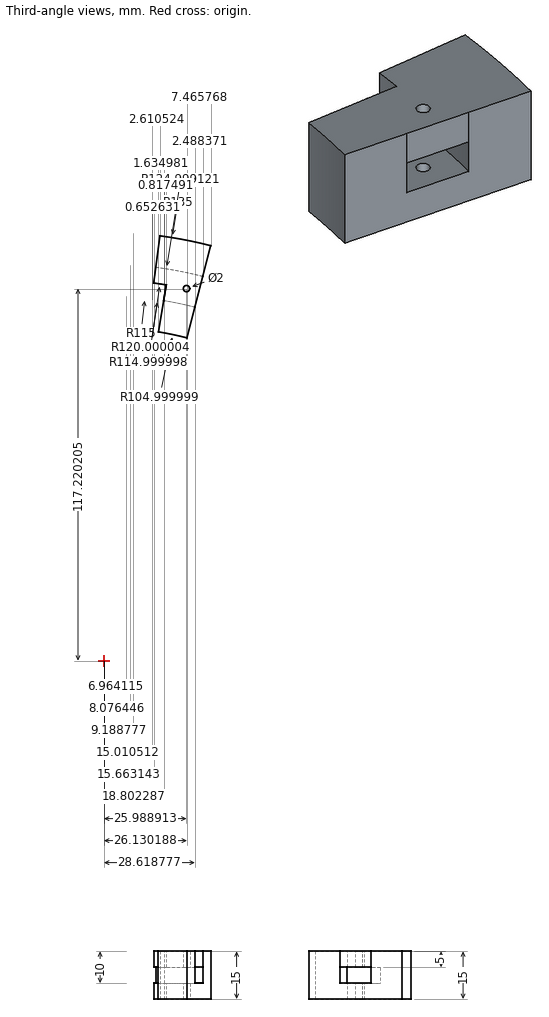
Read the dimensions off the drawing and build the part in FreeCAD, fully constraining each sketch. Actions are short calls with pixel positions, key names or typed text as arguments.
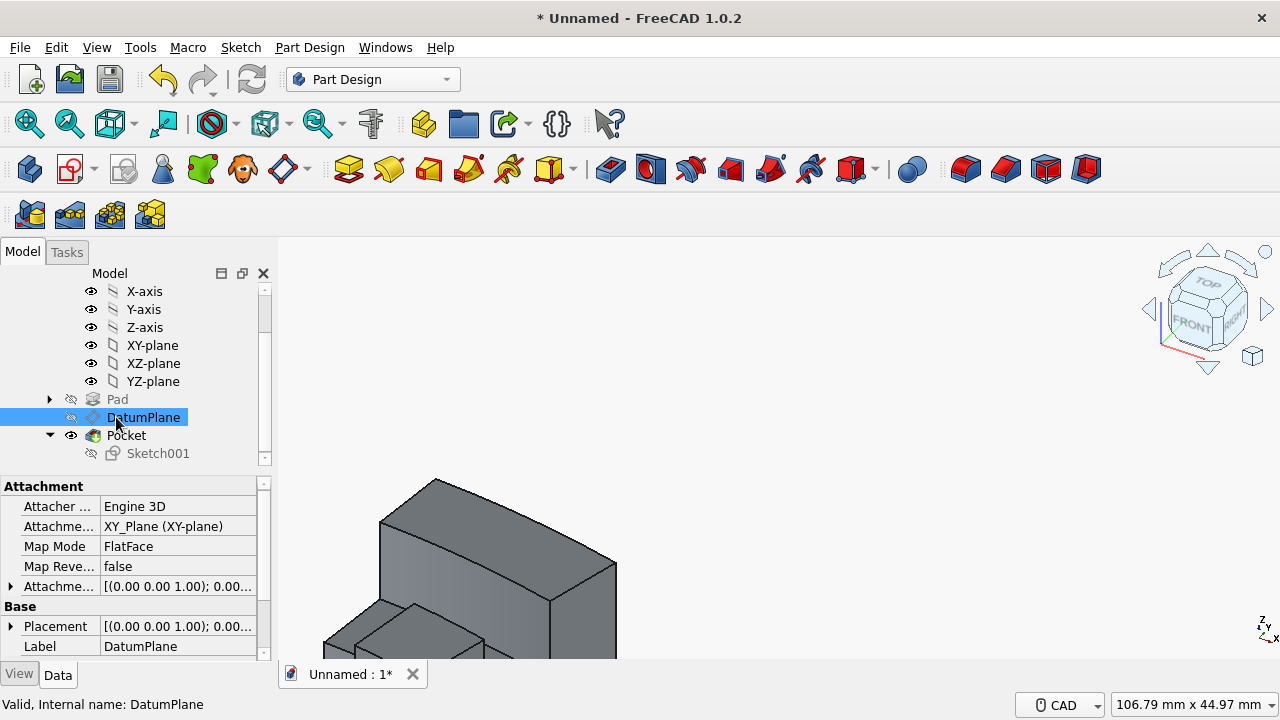
click(30, 124)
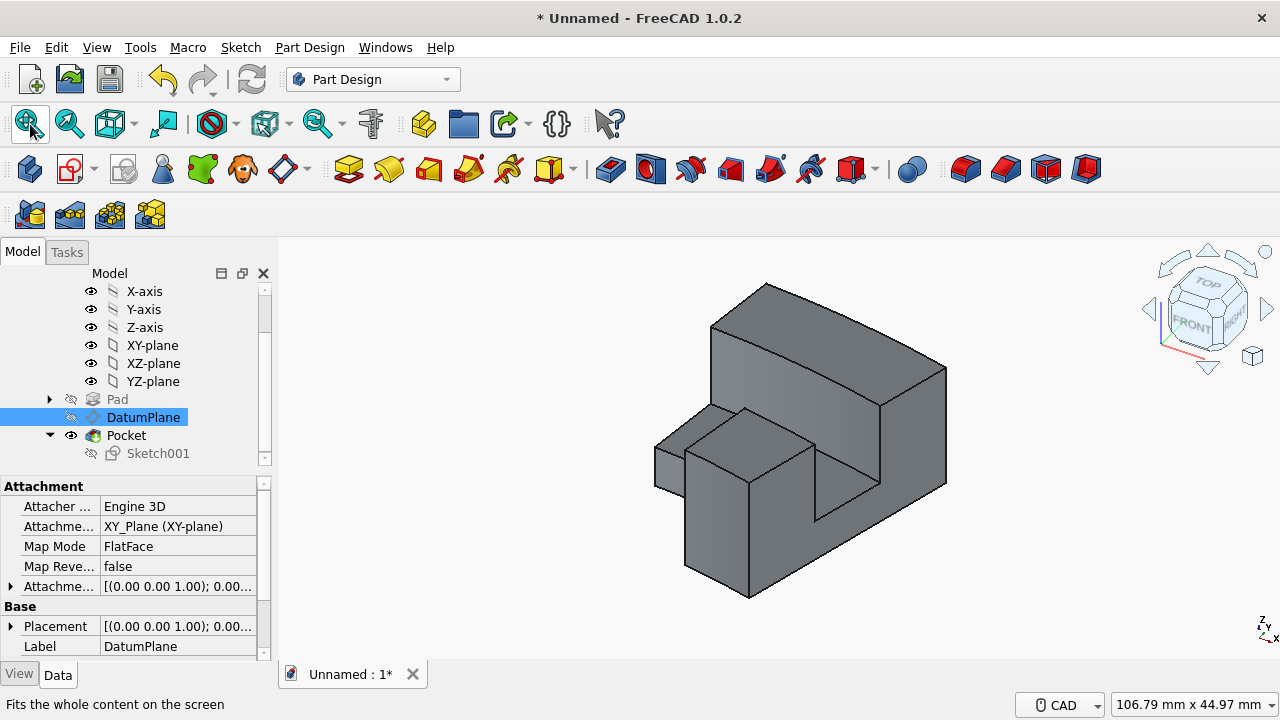
scroll(160, 377, down, 3)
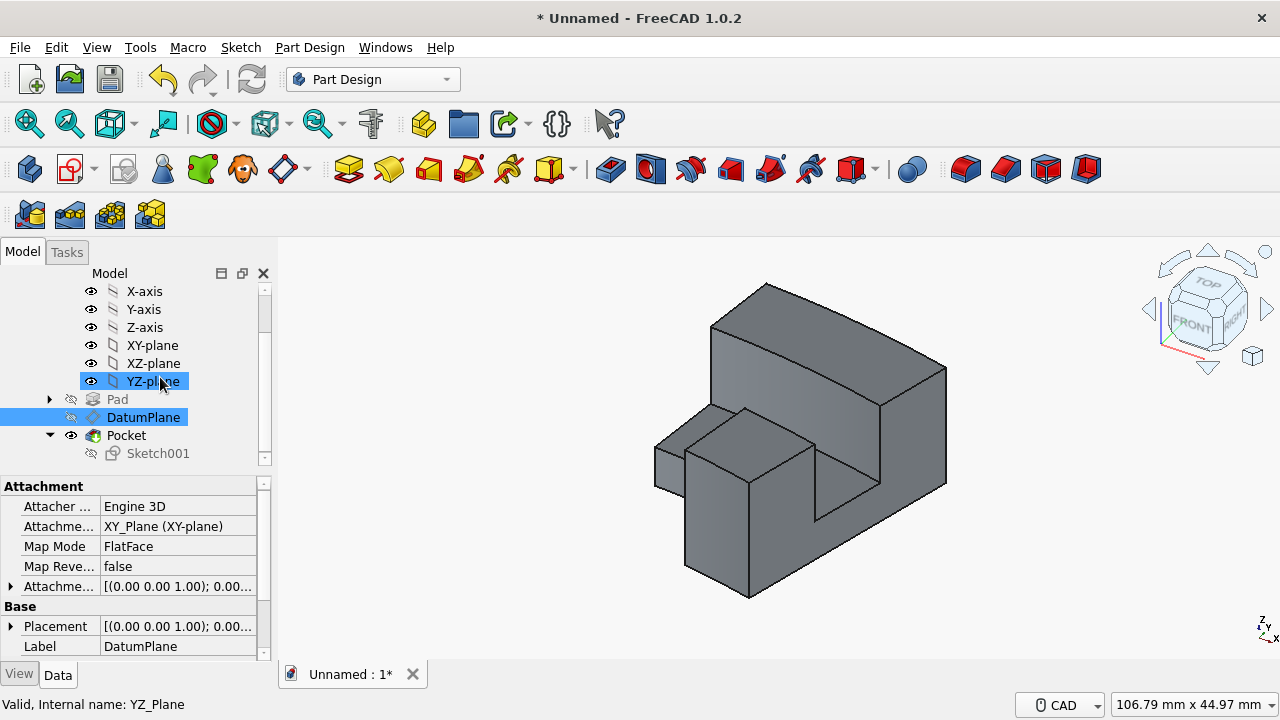
scroll(160, 377, up, 15)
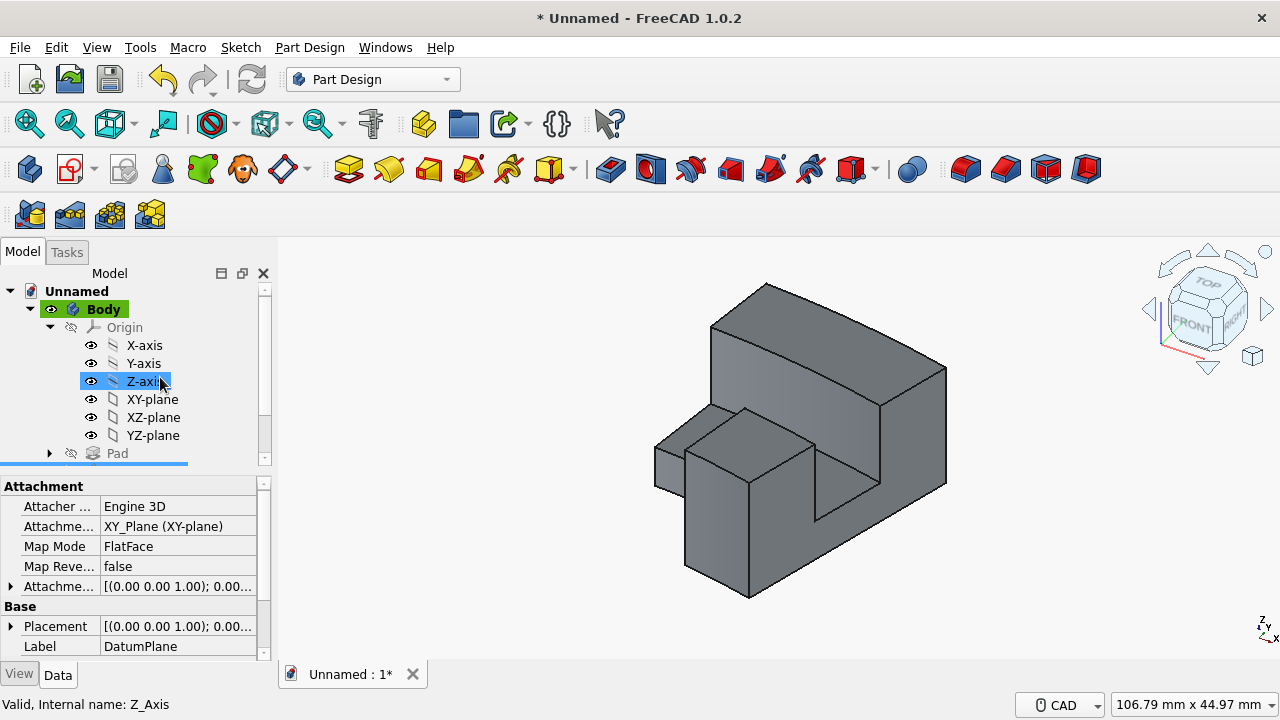
click(136, 399)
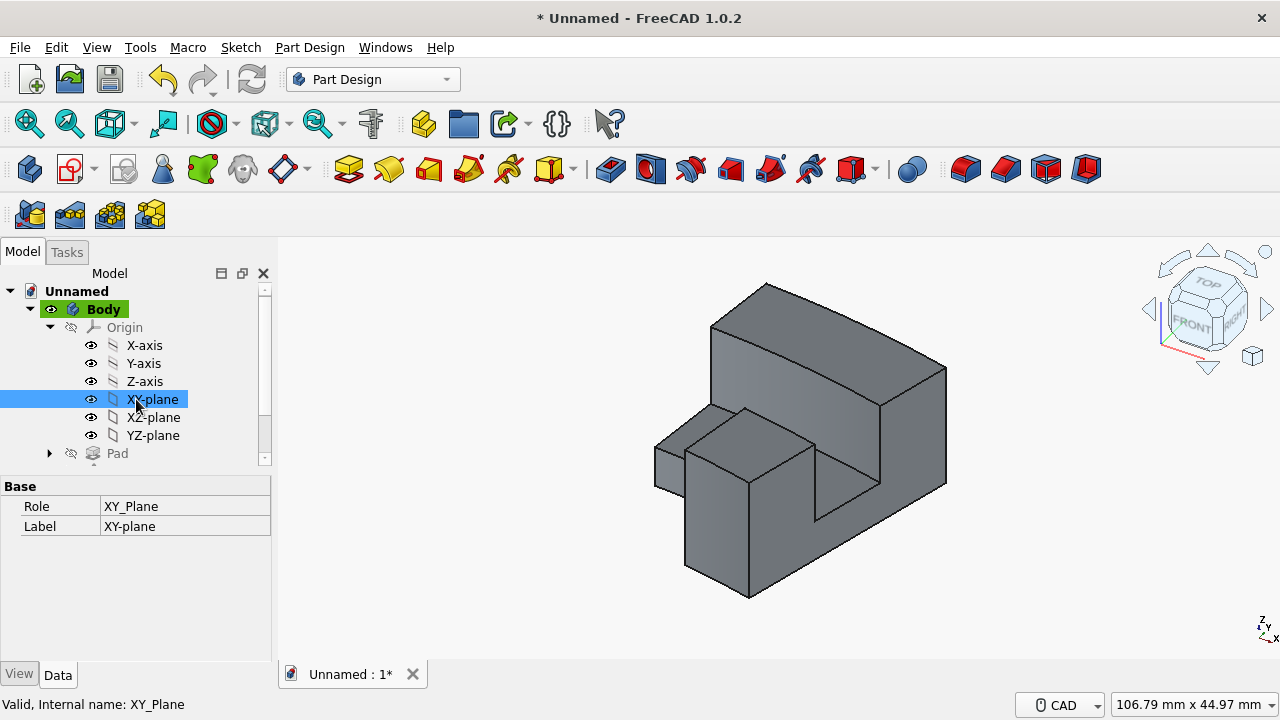
click(284, 170)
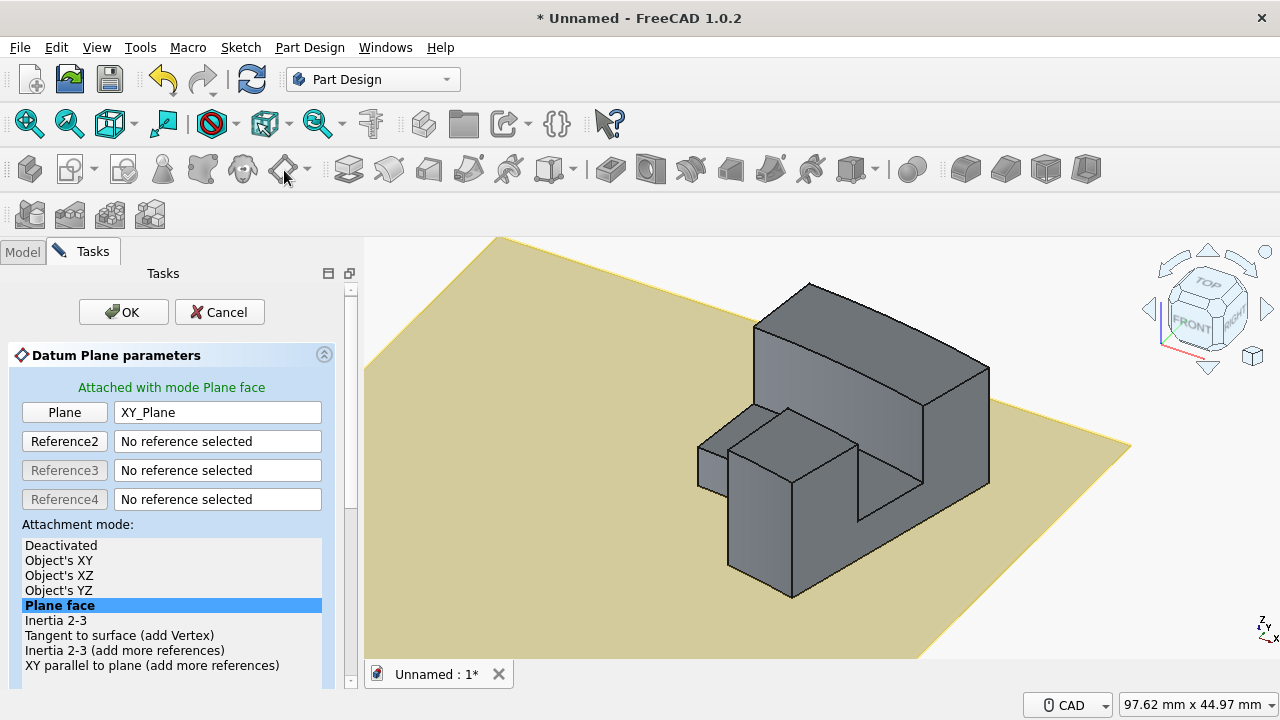
scroll(351, 486, down, 4)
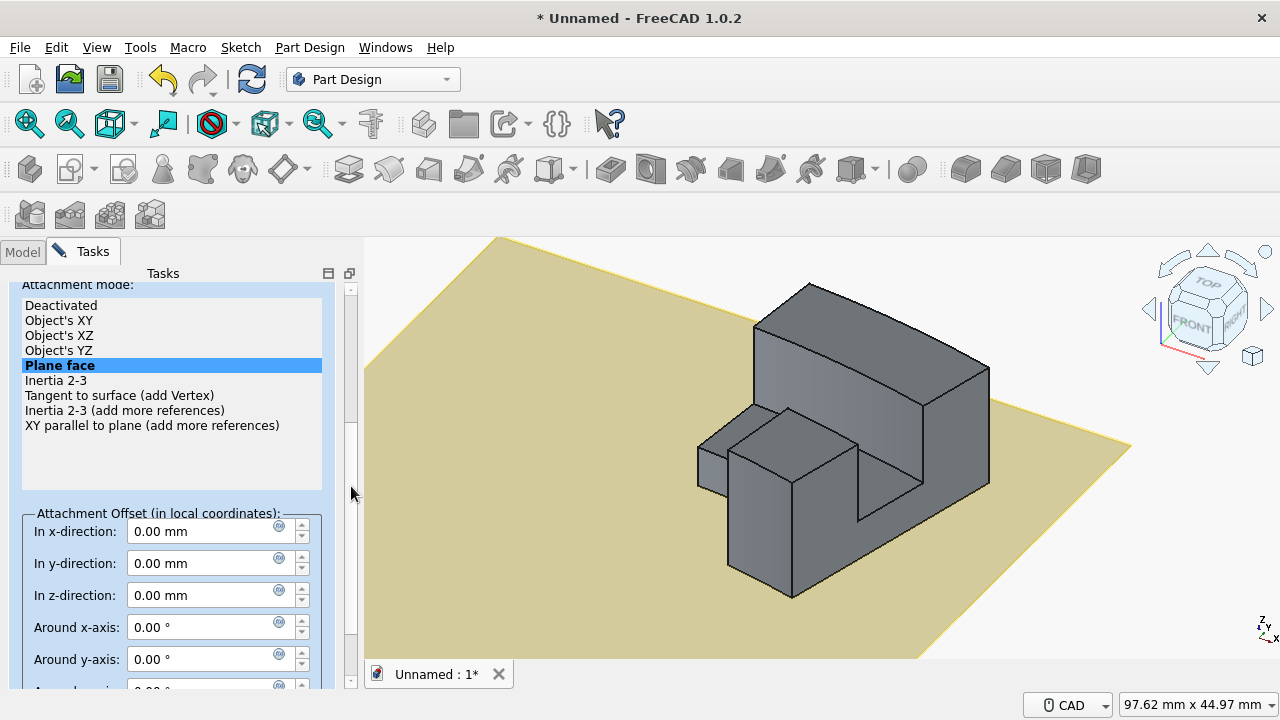
triple_click(210, 595)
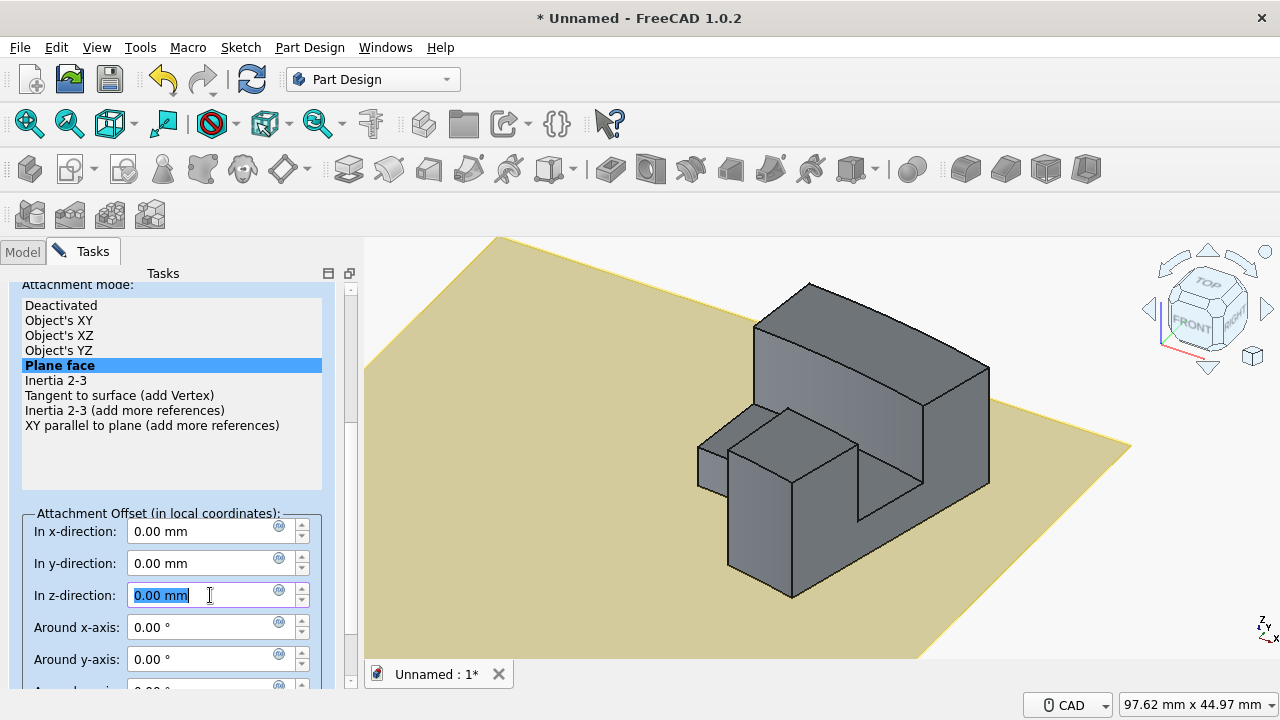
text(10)
key(Tab)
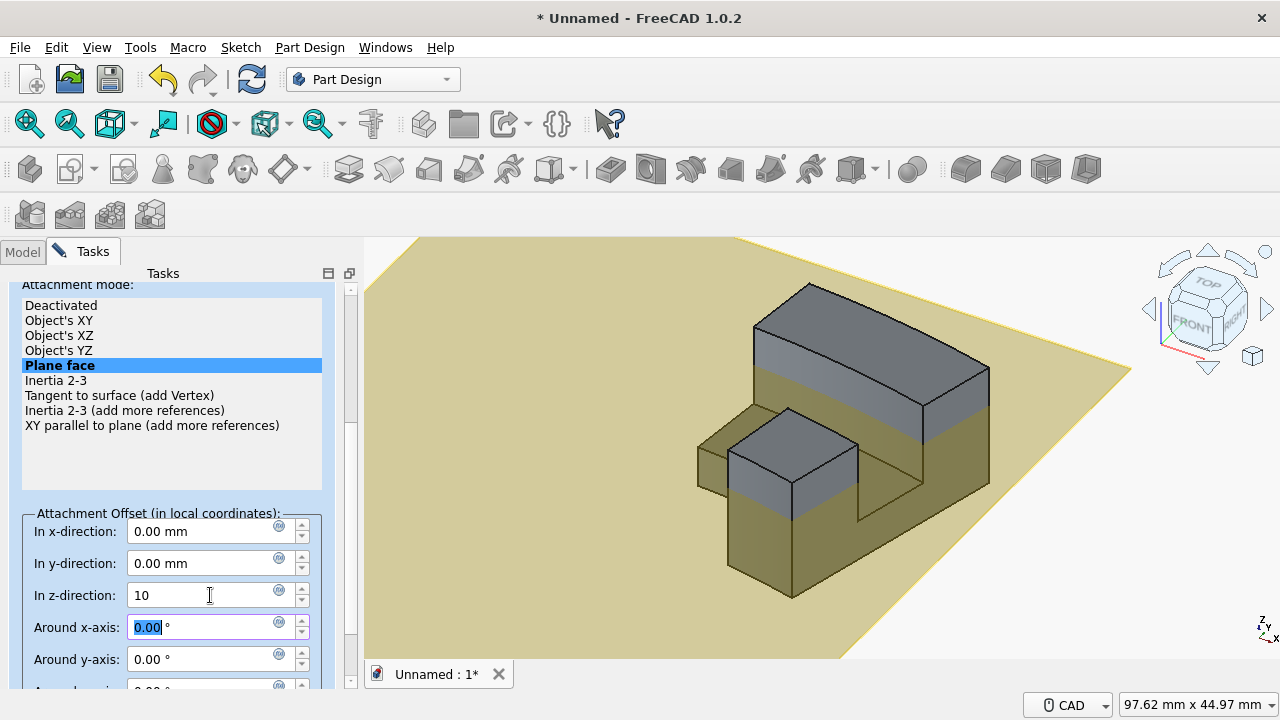
scroll(351, 486, up, 5)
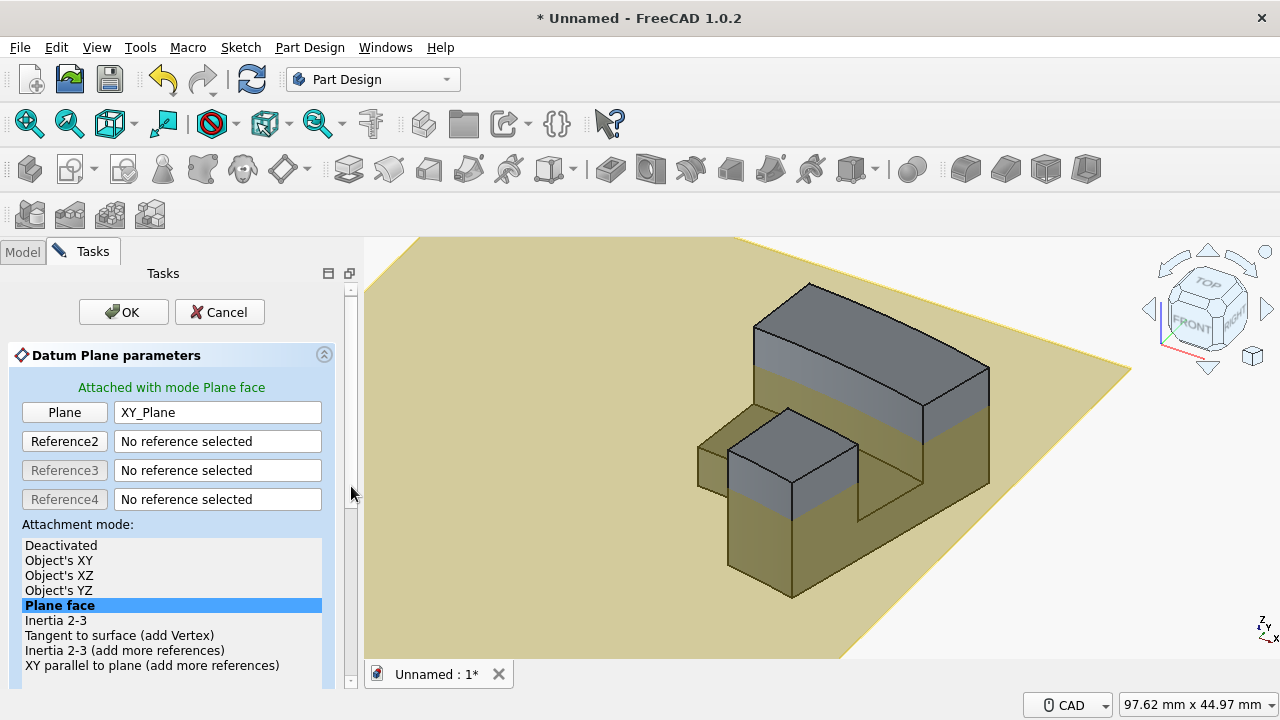
click(124, 312)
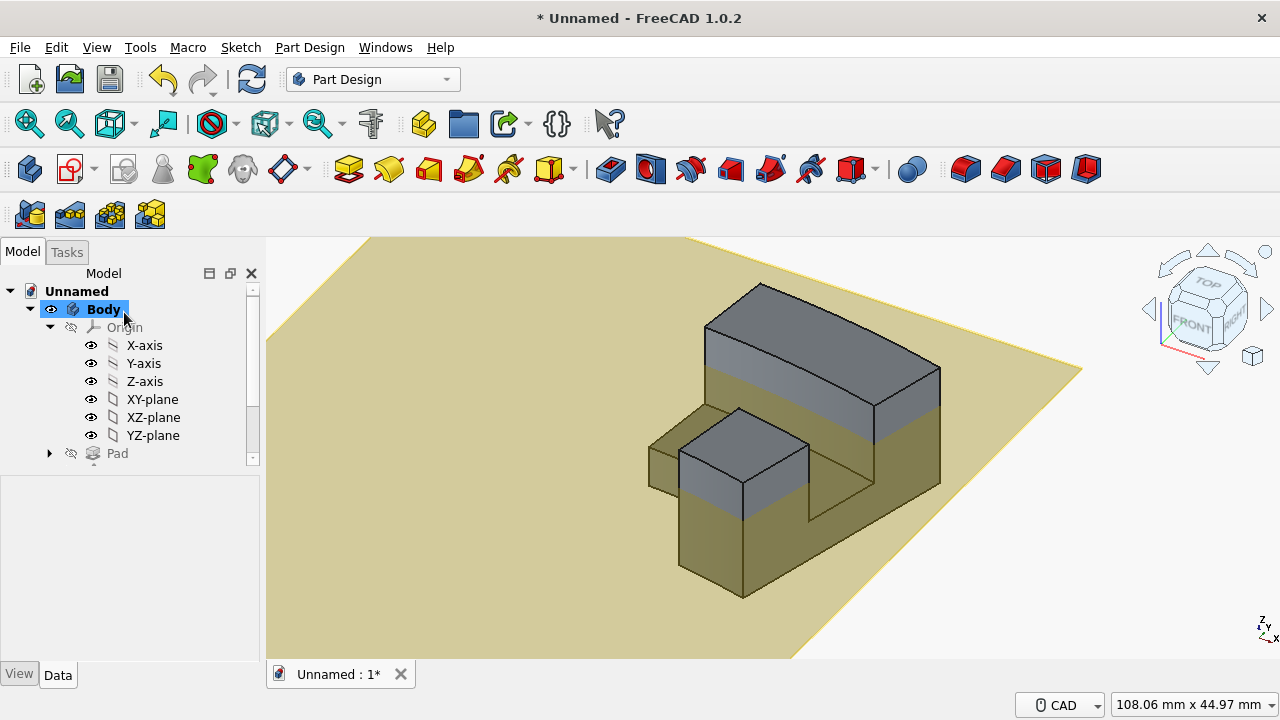
scroll(100, 377, down, 3)